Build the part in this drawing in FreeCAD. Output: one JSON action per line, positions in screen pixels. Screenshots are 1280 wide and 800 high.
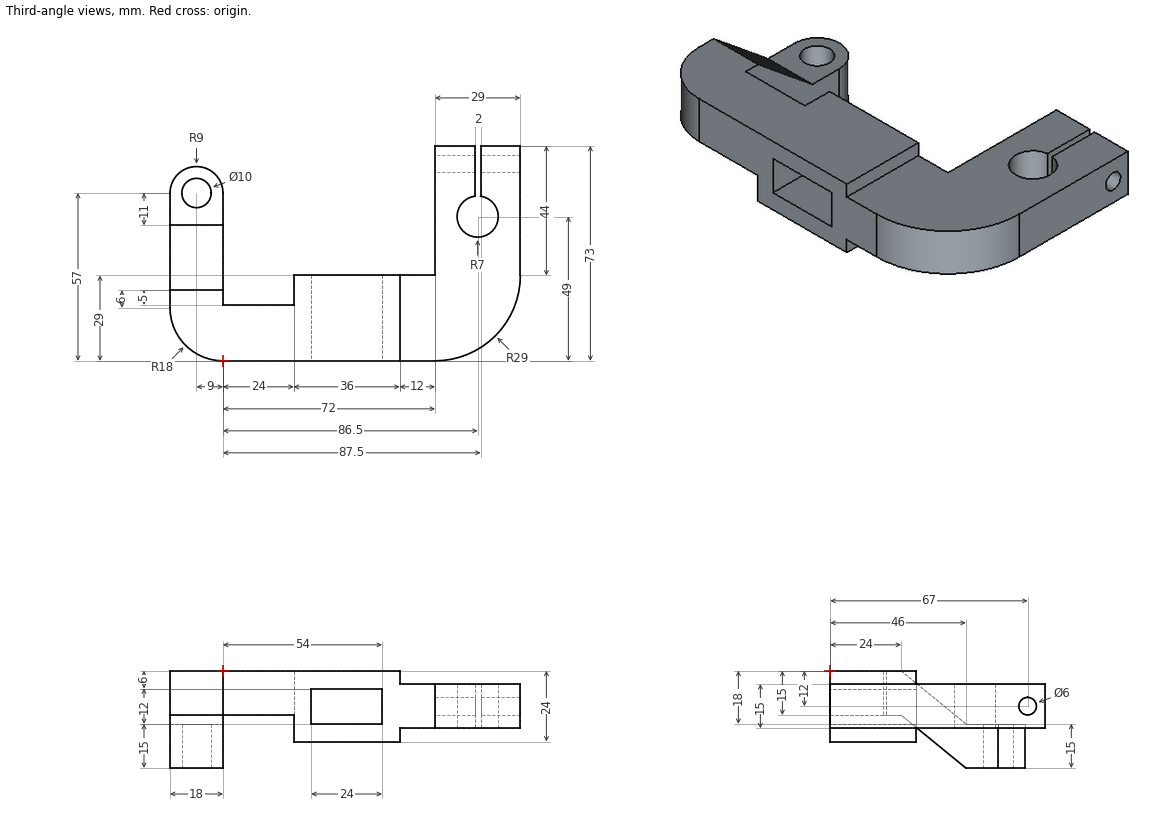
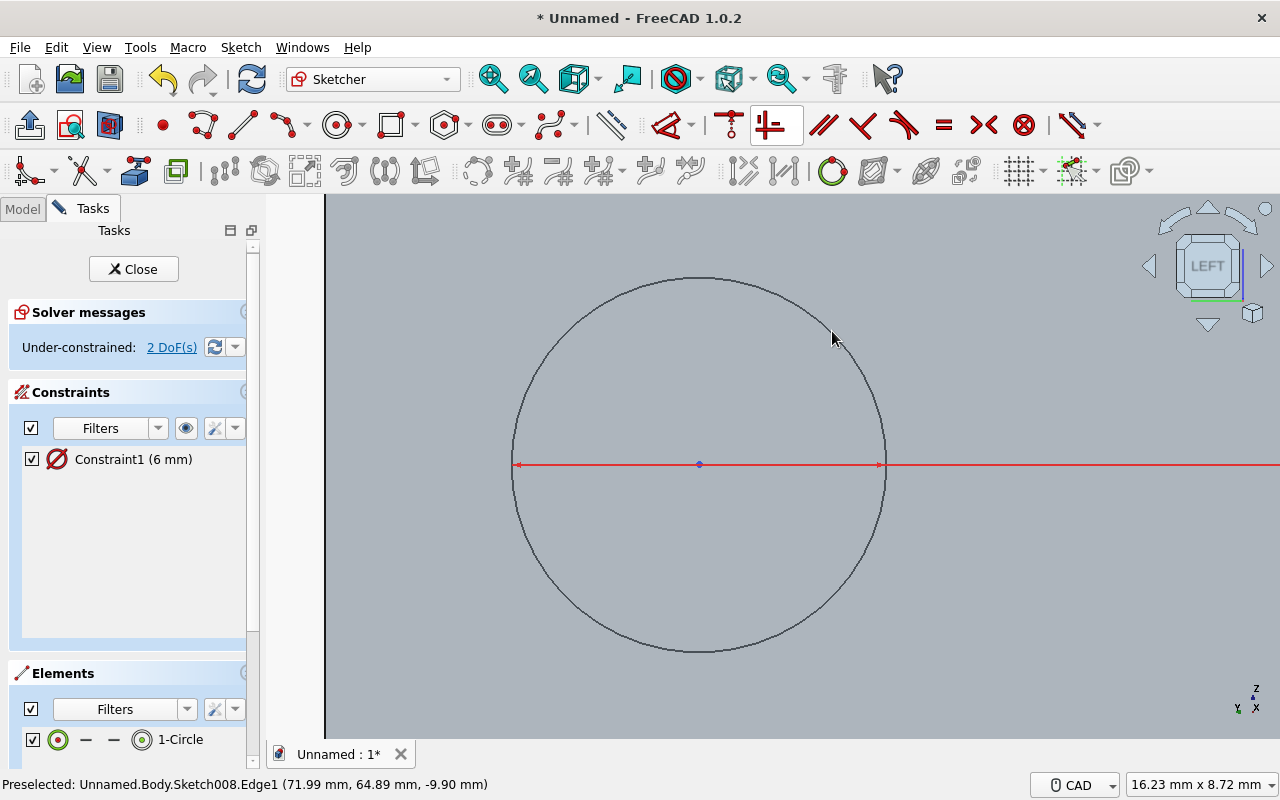
{"action": "left_click", "coordinate": [666, 126]}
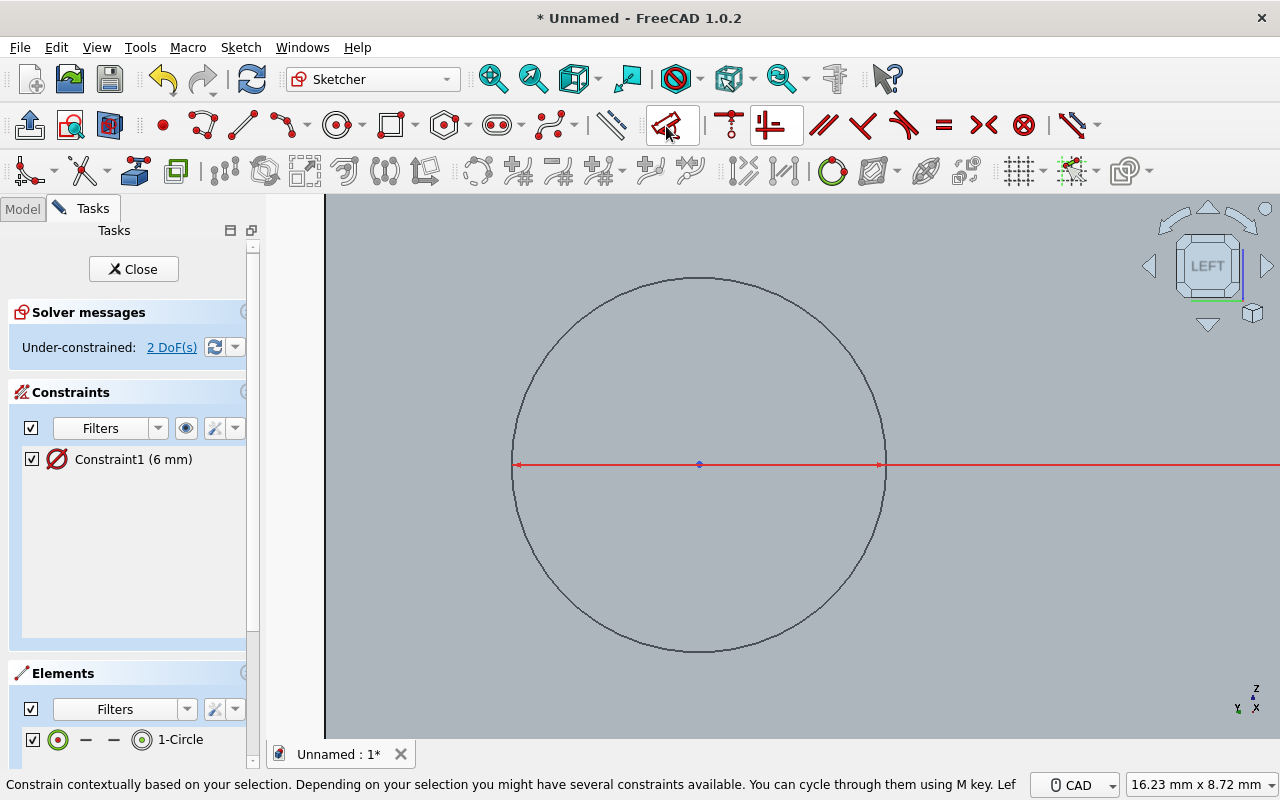
{"action": "left_click", "coordinate": [699, 465]}
{"action": "left_click", "coordinate": [907, 499]}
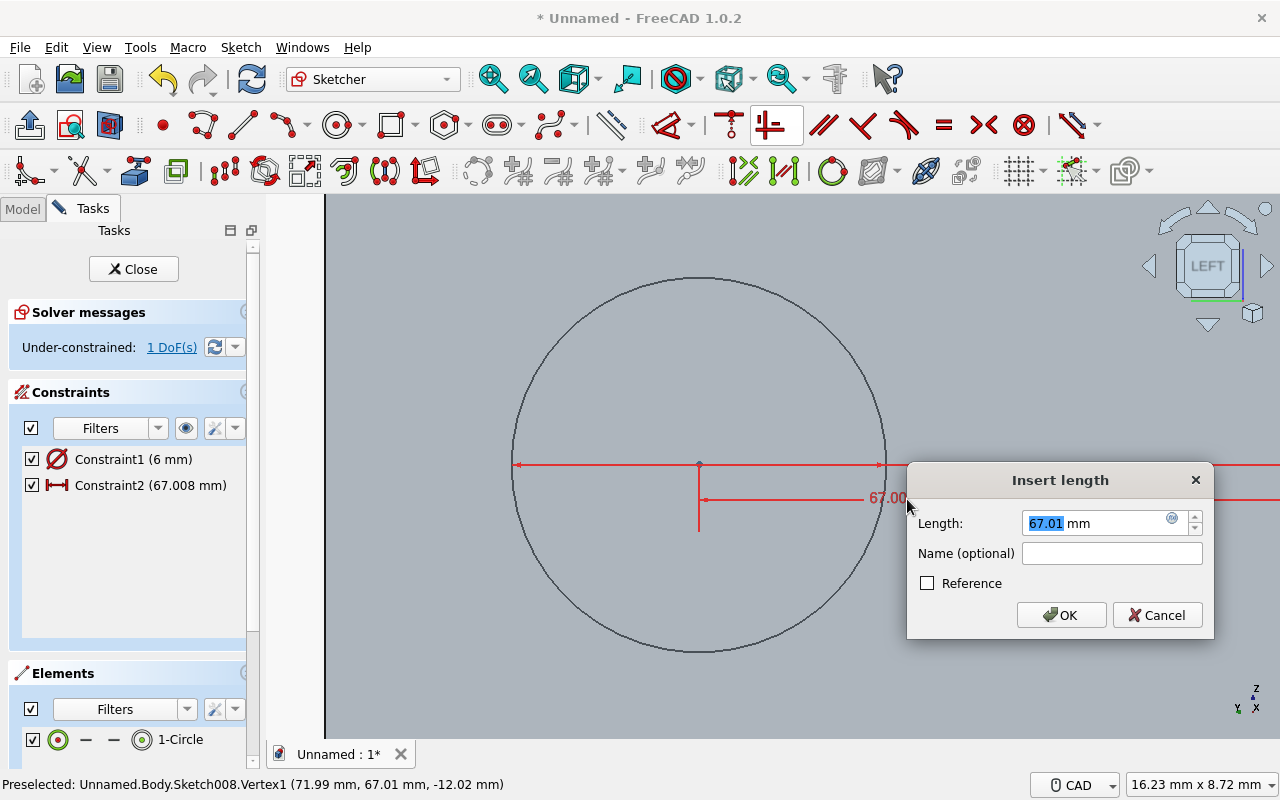
{"action": "type", "text": "67"}
{"action": "key", "text": "Return"}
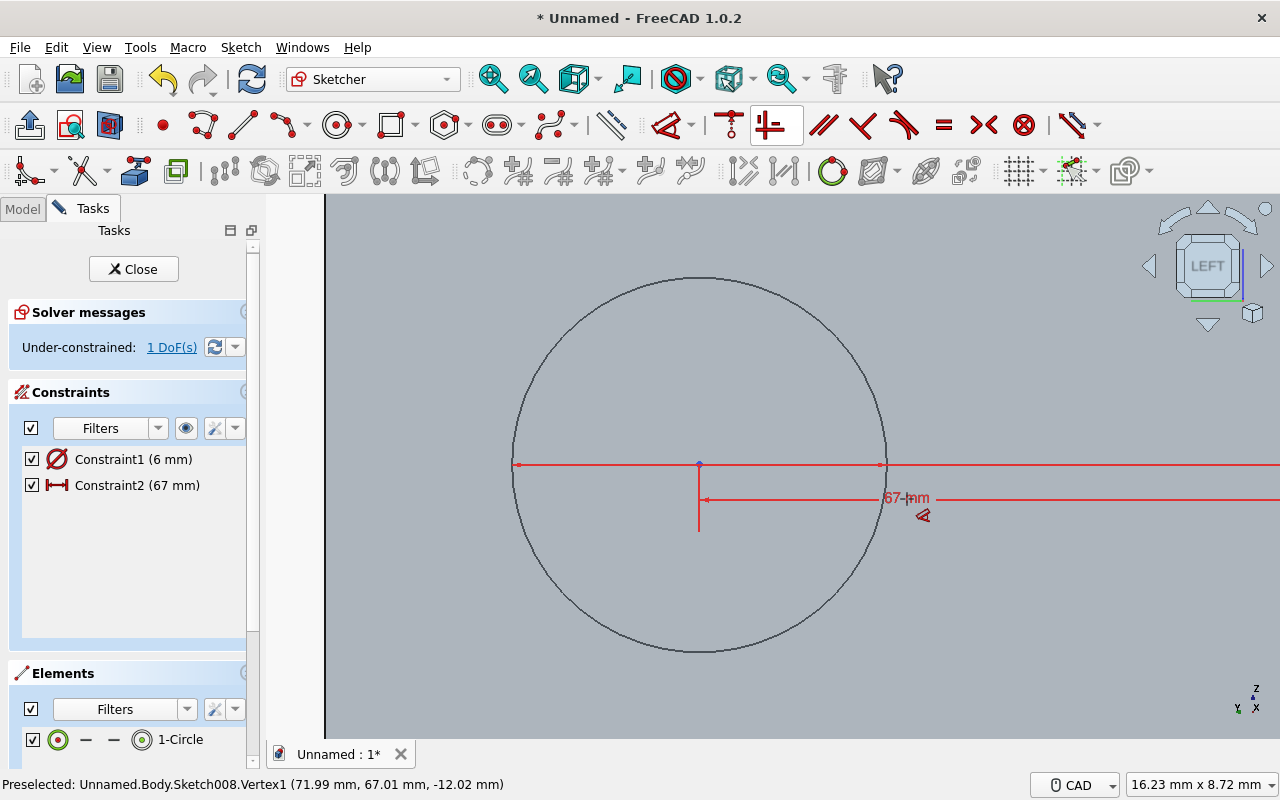
{"action": "left_click", "coordinate": [699, 465]}
{"action": "left_click", "coordinate": [665, 343]}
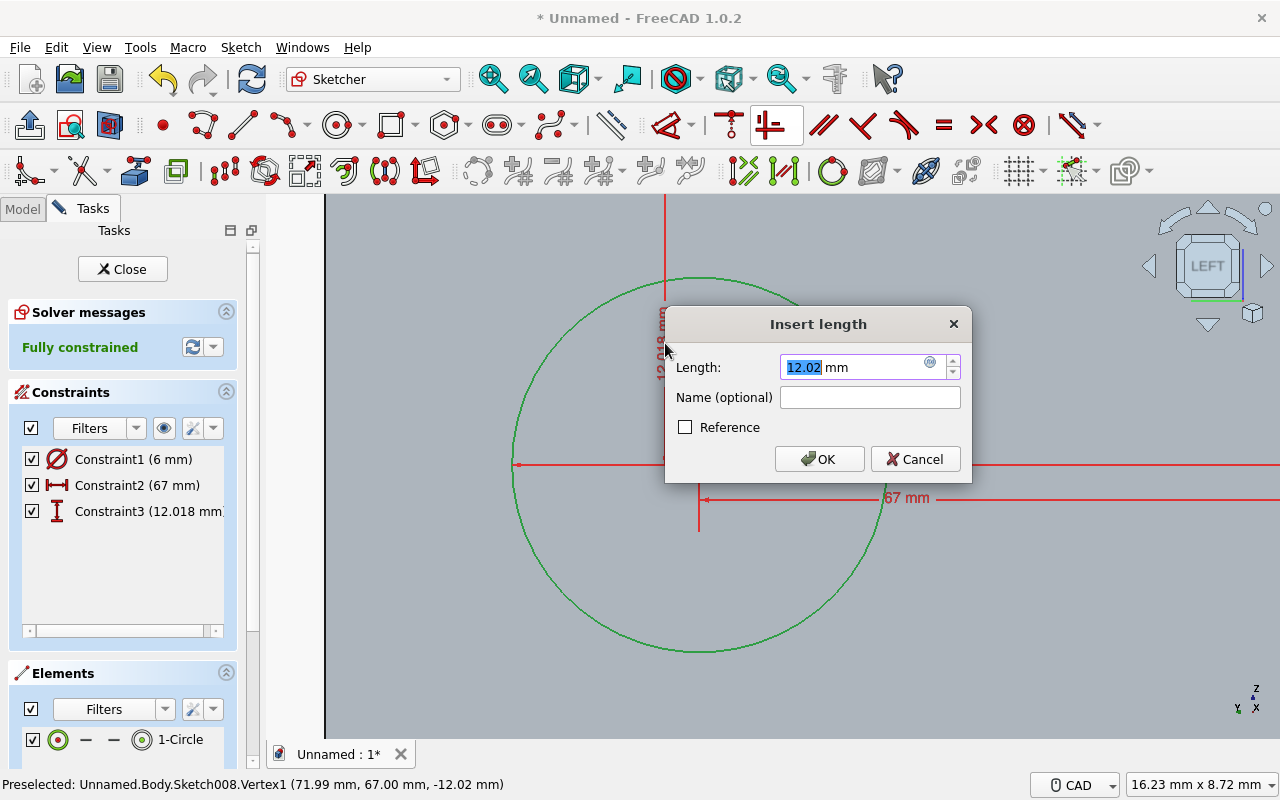
{"action": "type", "text": "12"}
{"action": "key", "text": "Return"}
{"action": "key", "text": "Escape"}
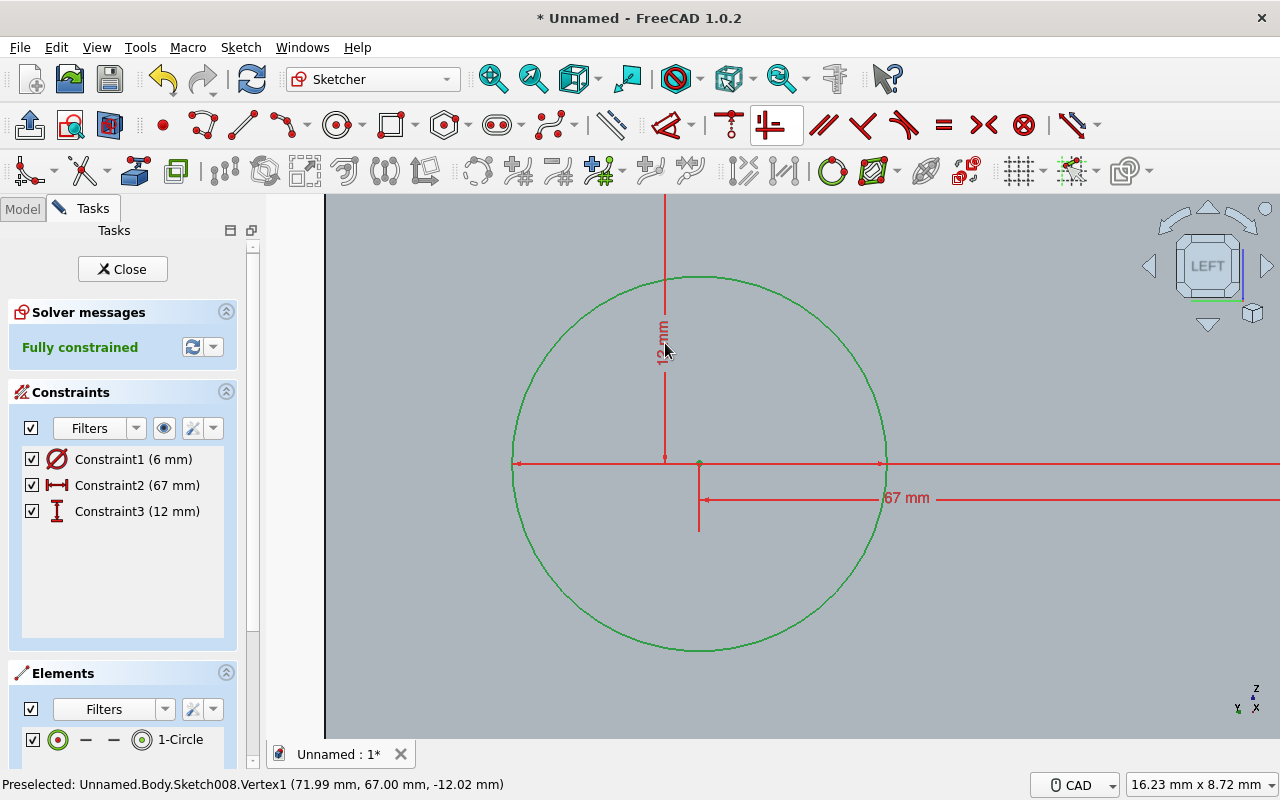
{"action": "left_click", "coordinate": [123, 269]}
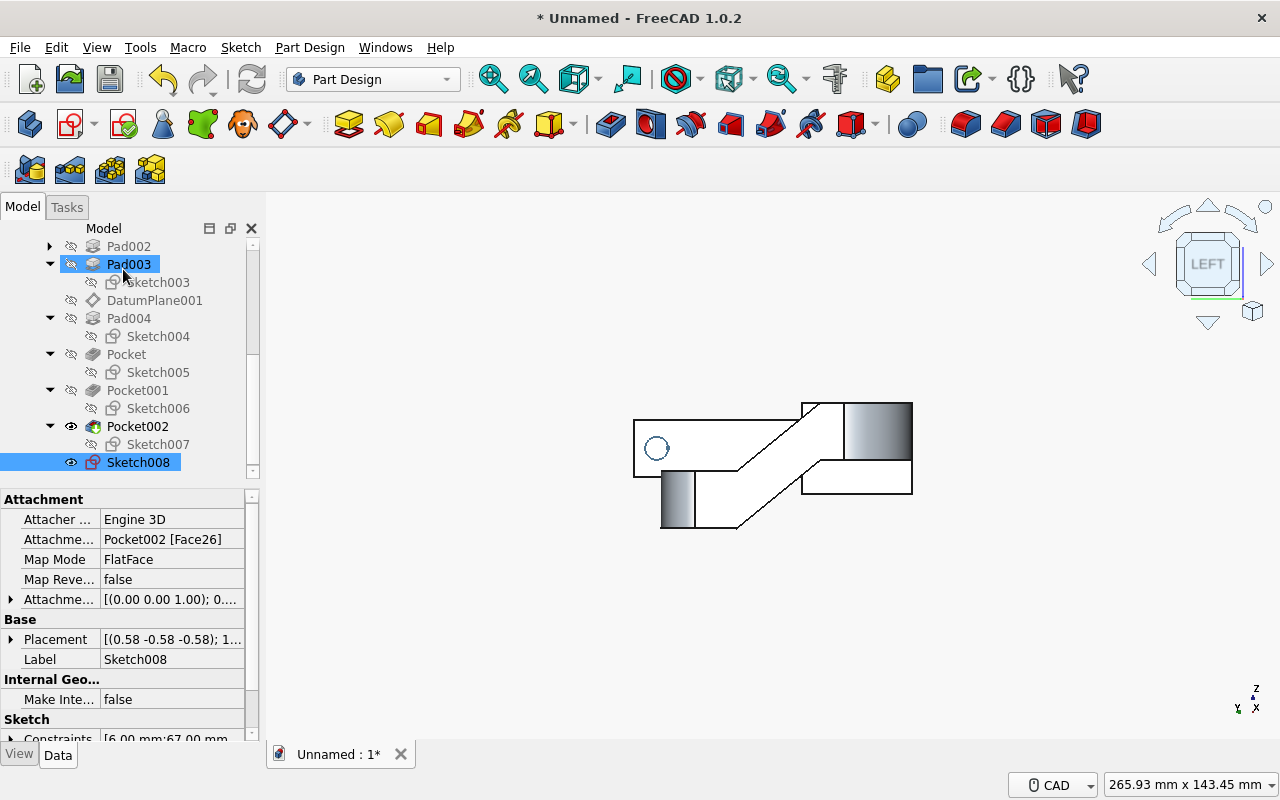
{"action": "left_click", "coordinate": [612, 124]}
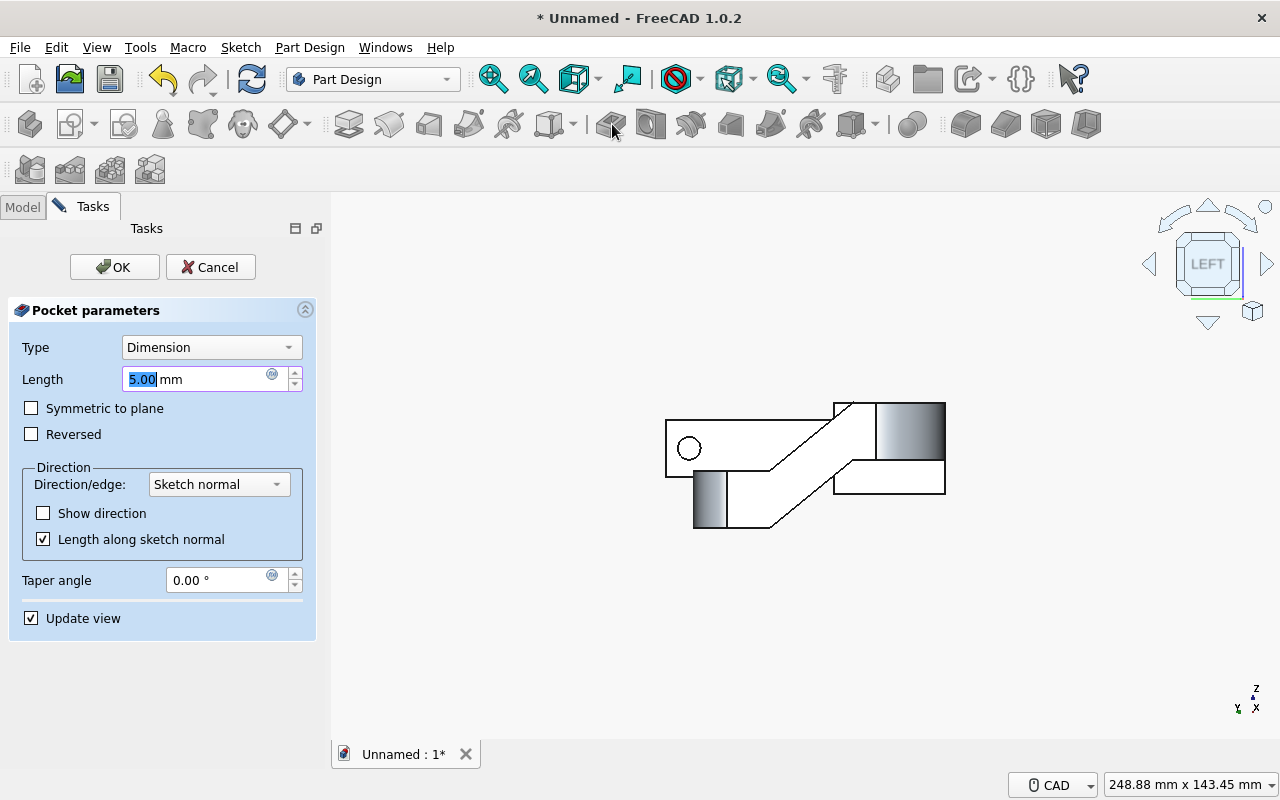
{"action": "left_click", "coordinate": [212, 348]}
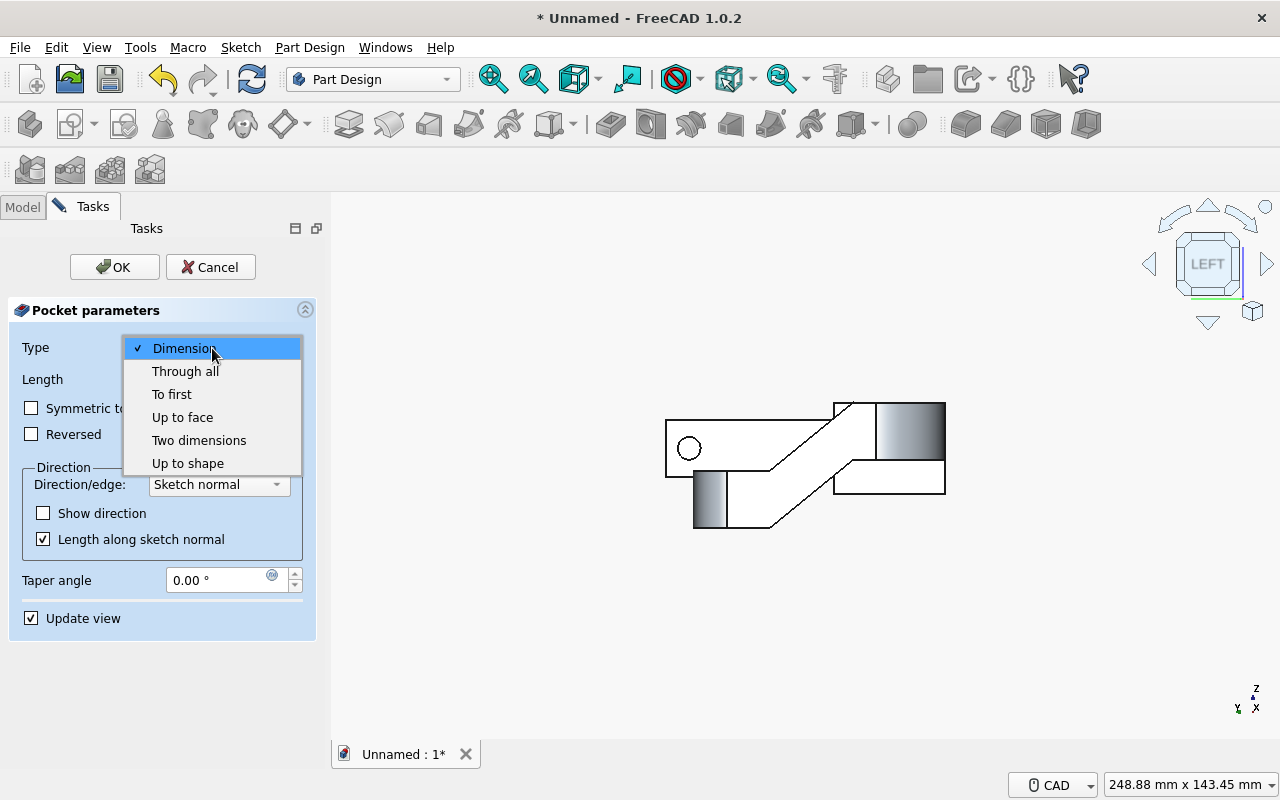
{"action": "left_click", "coordinate": [212, 372]}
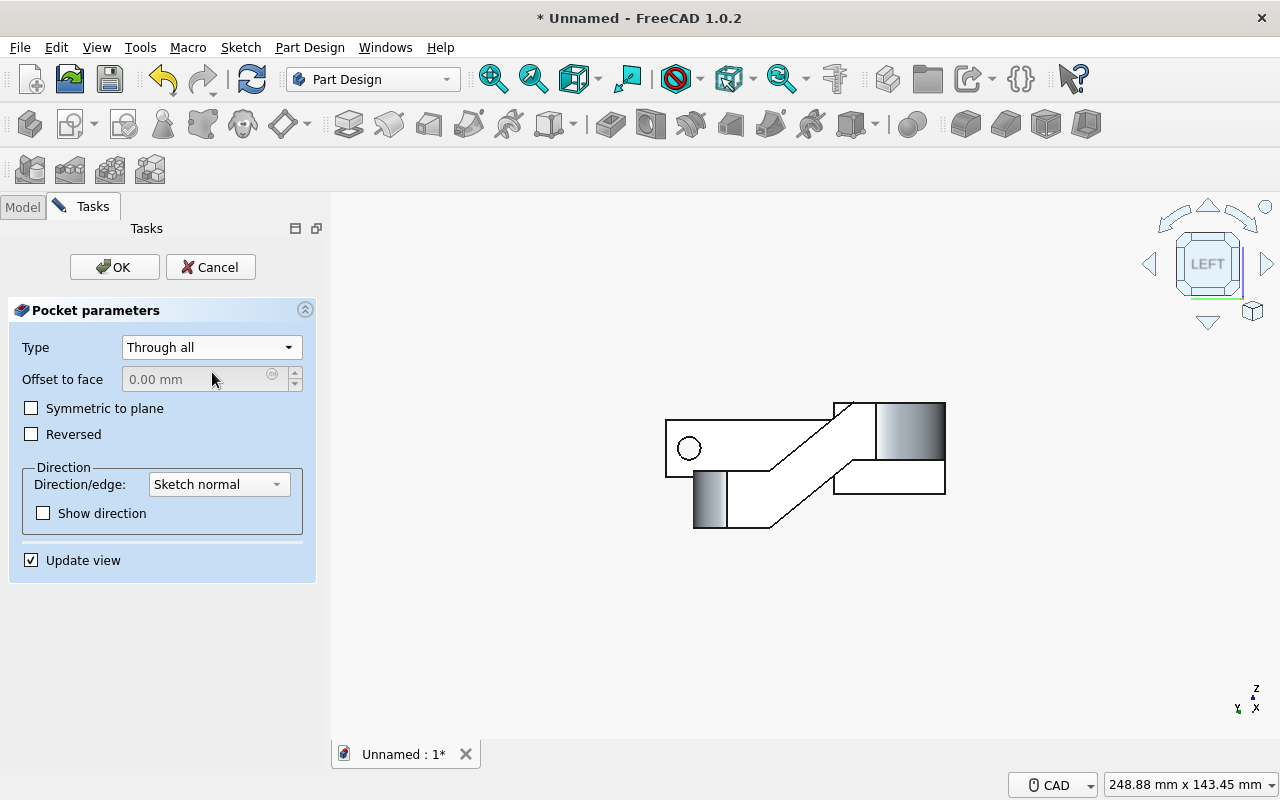
{"action": "left_click", "coordinate": [115, 267]}